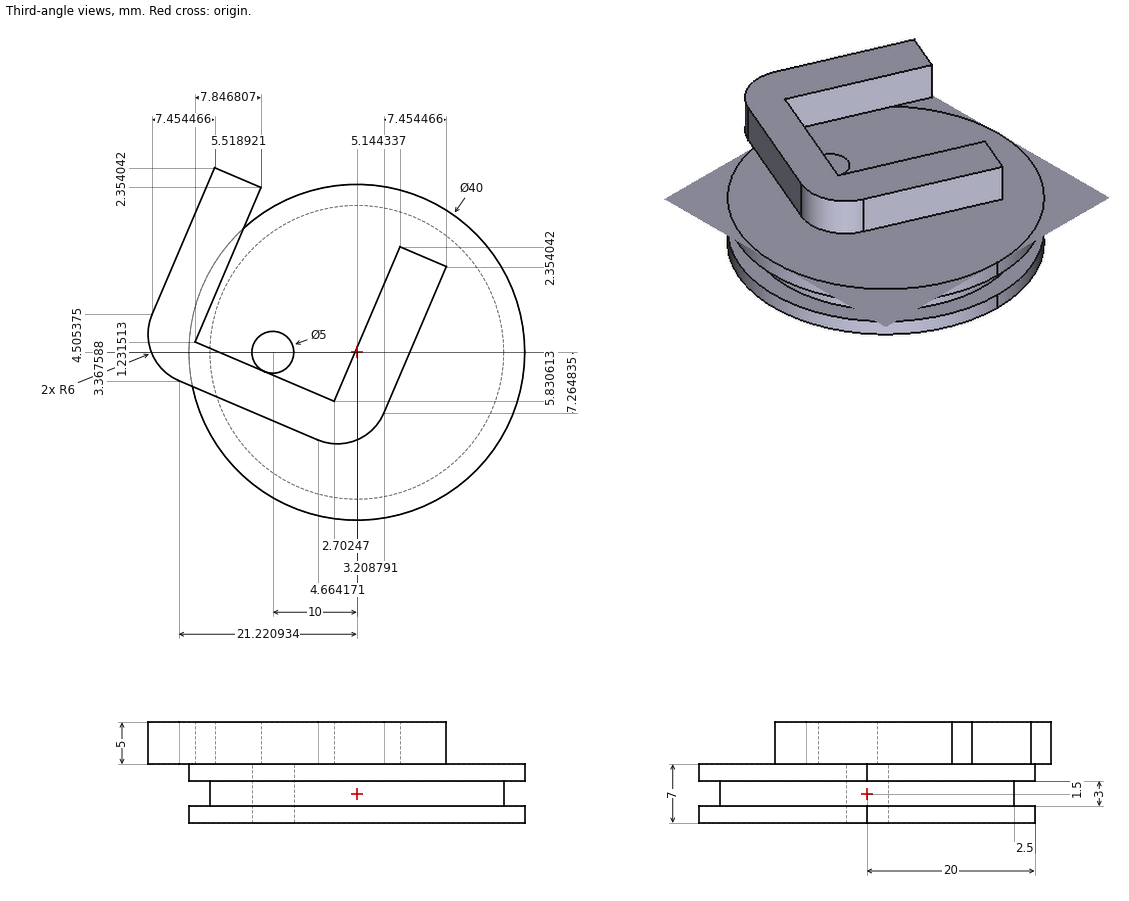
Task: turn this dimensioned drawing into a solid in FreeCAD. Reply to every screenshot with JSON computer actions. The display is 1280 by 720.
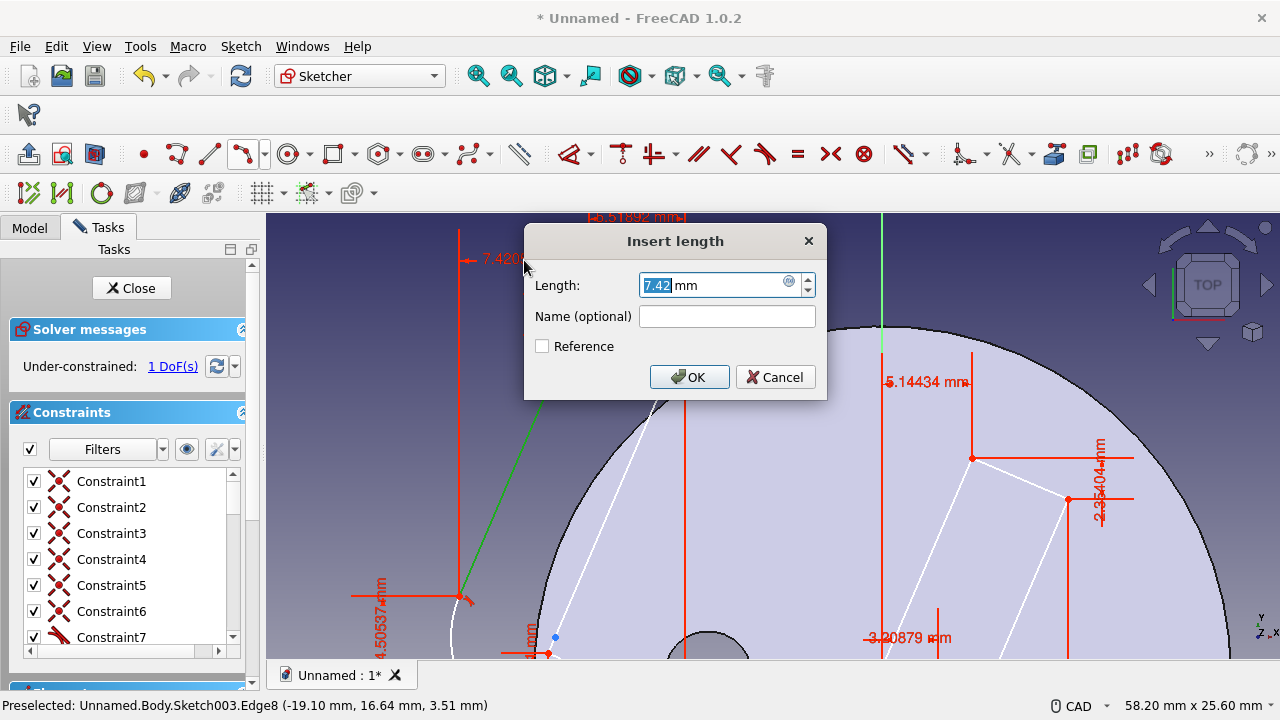
{"action": "type", "text": "7.454466"}
{"action": "key", "text": "Return"}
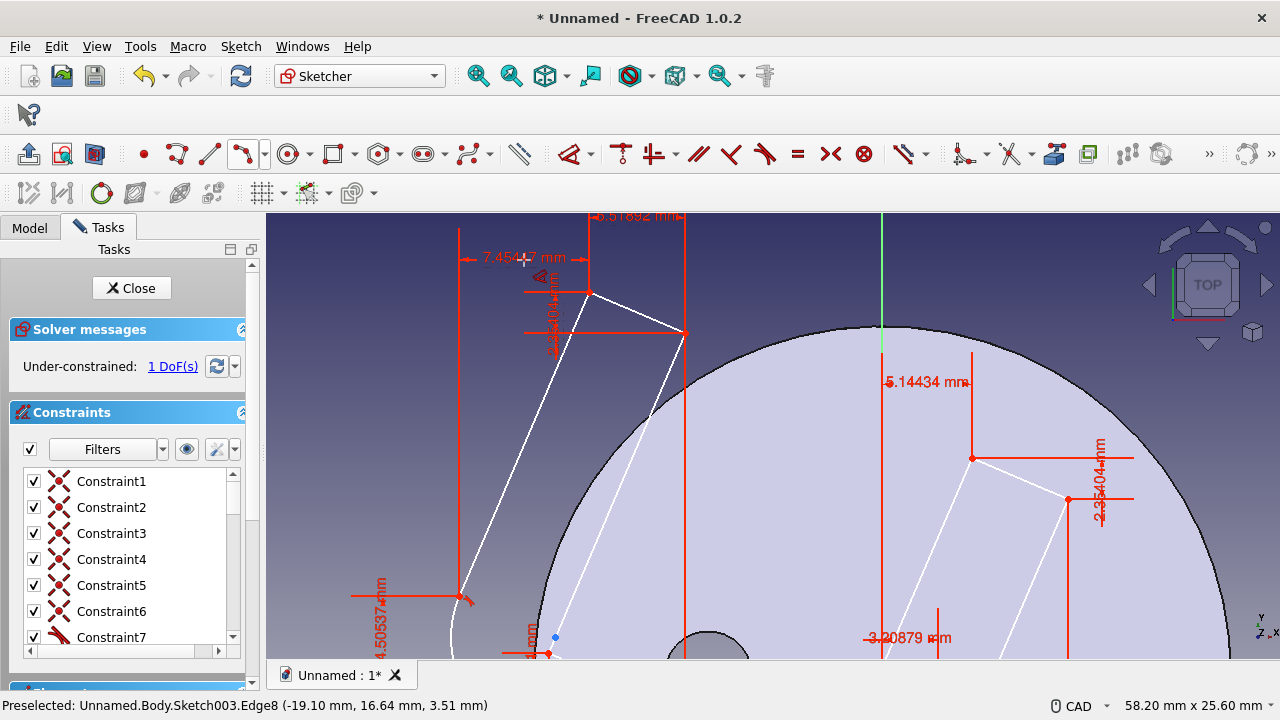
{"action": "scroll", "coordinate": [657, 323], "scroll_direction": "down", "scroll_amount": 4}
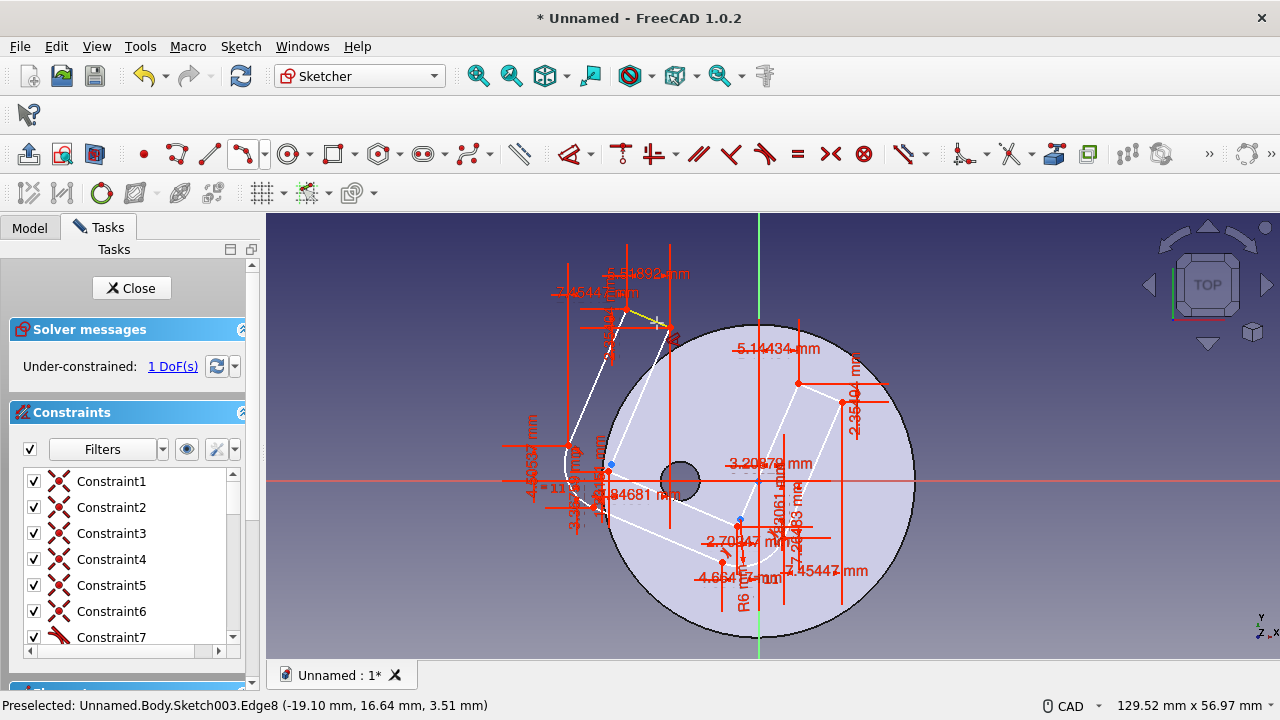
{"action": "left_click", "coordinate": [593, 508]}
{"action": "left_click", "coordinate": [638, 542]}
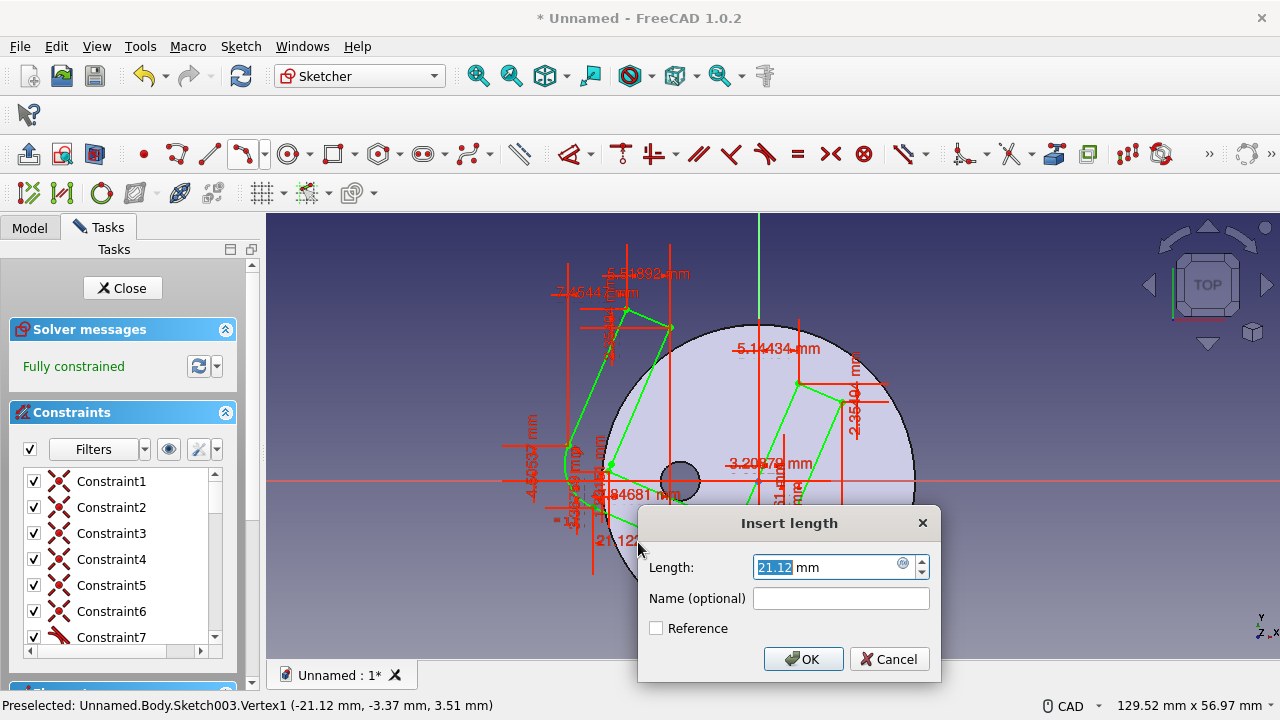
{"action": "type", "text": "21.220934"}
{"action": "key", "text": "Return"}
{"action": "key", "text": "Escape"}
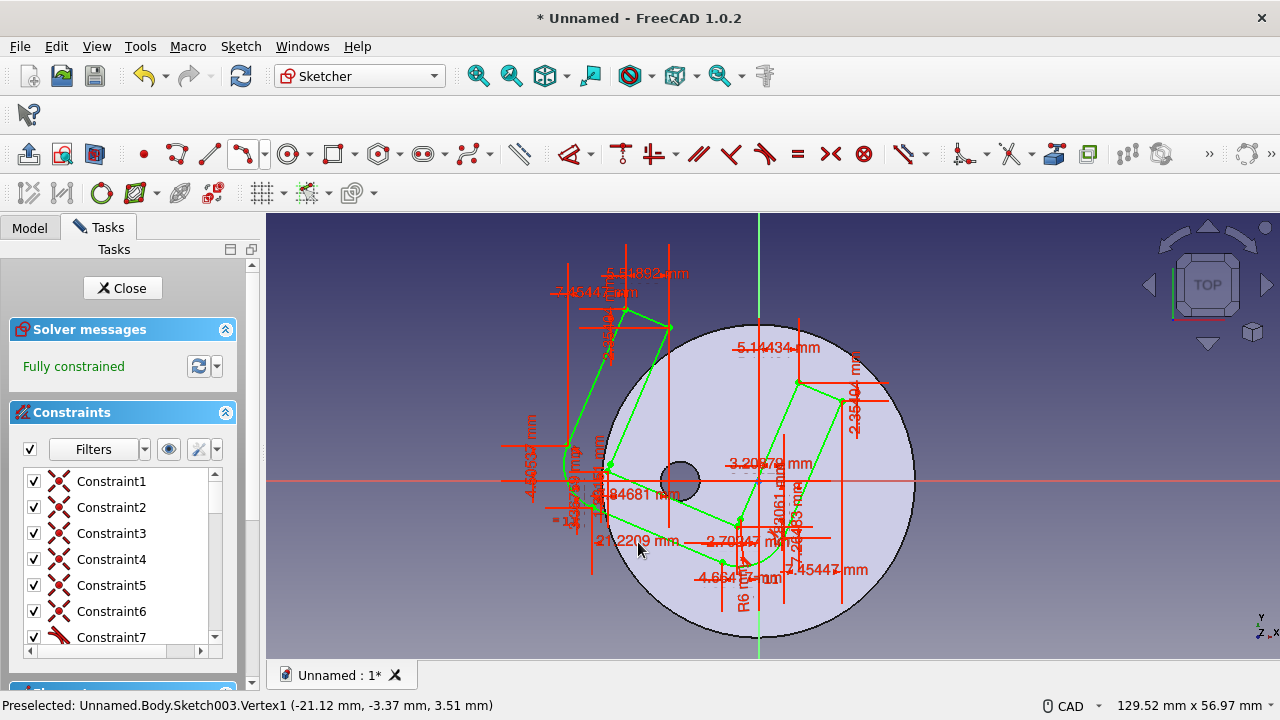
{"action": "left_click", "coordinate": [123, 288]}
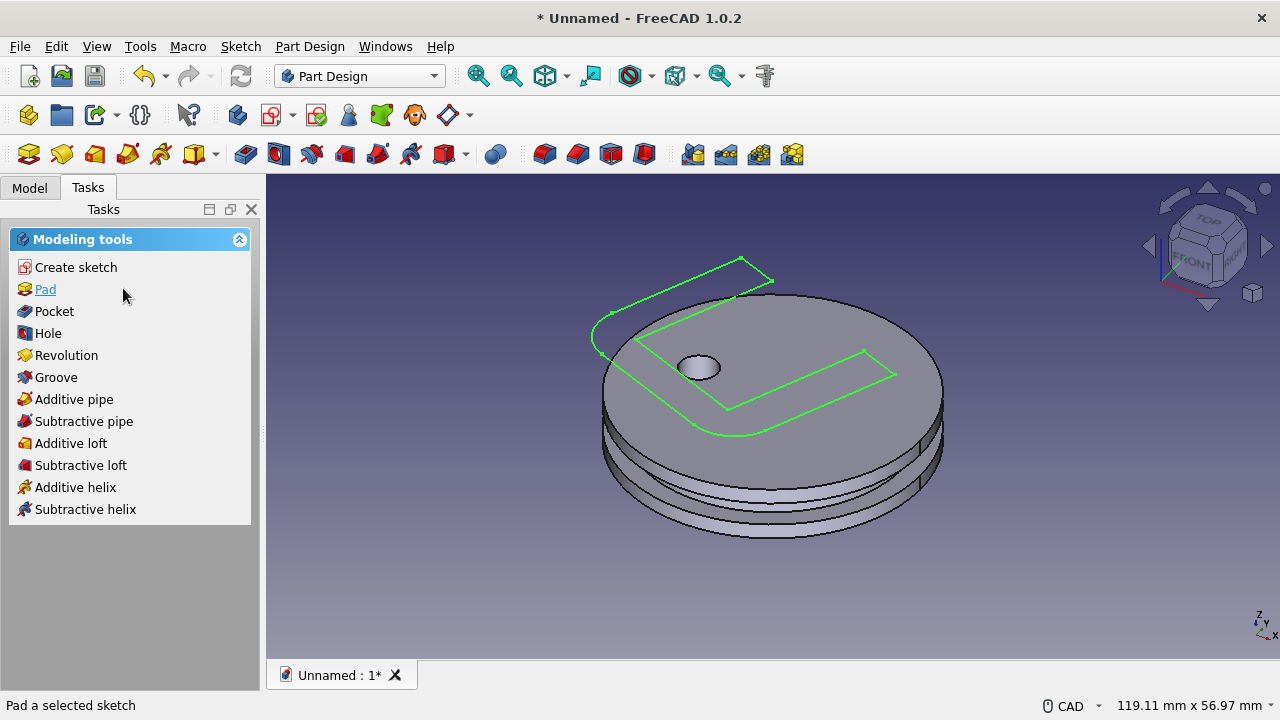
{"action": "left_click", "coordinate": [29, 154]}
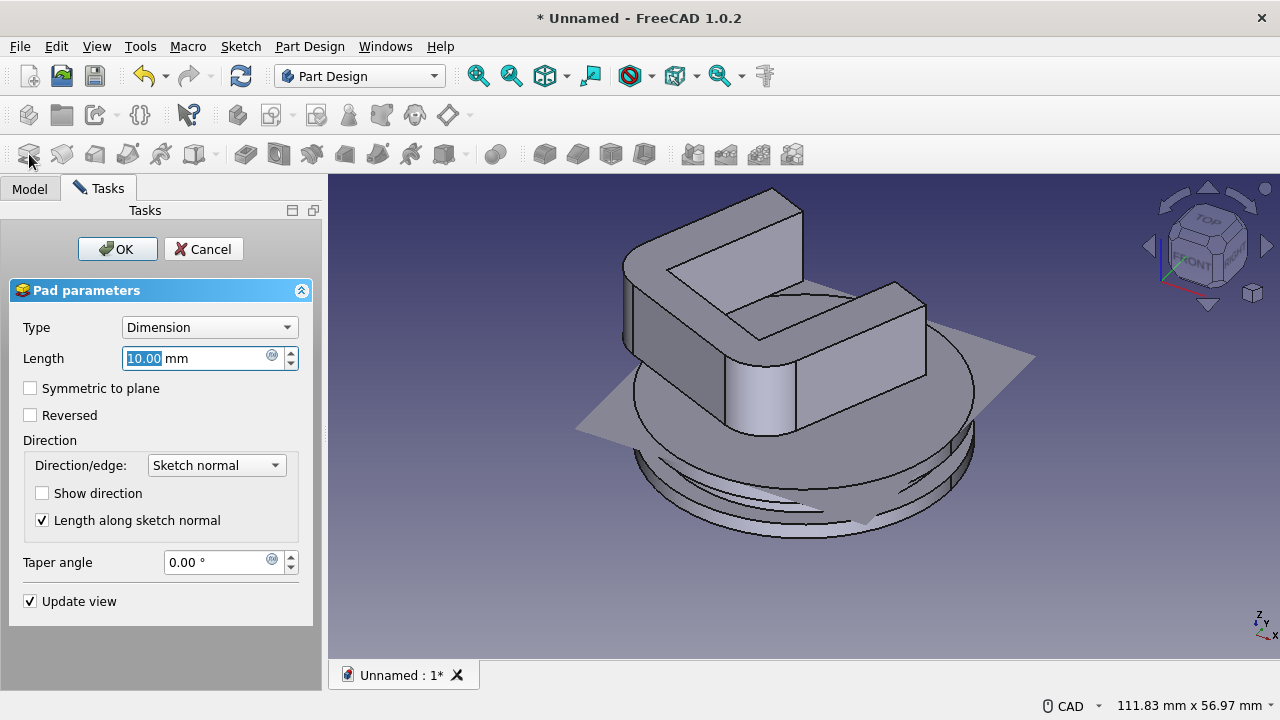
{"action": "type", "text": "5"}
{"action": "key", "text": "Tab"}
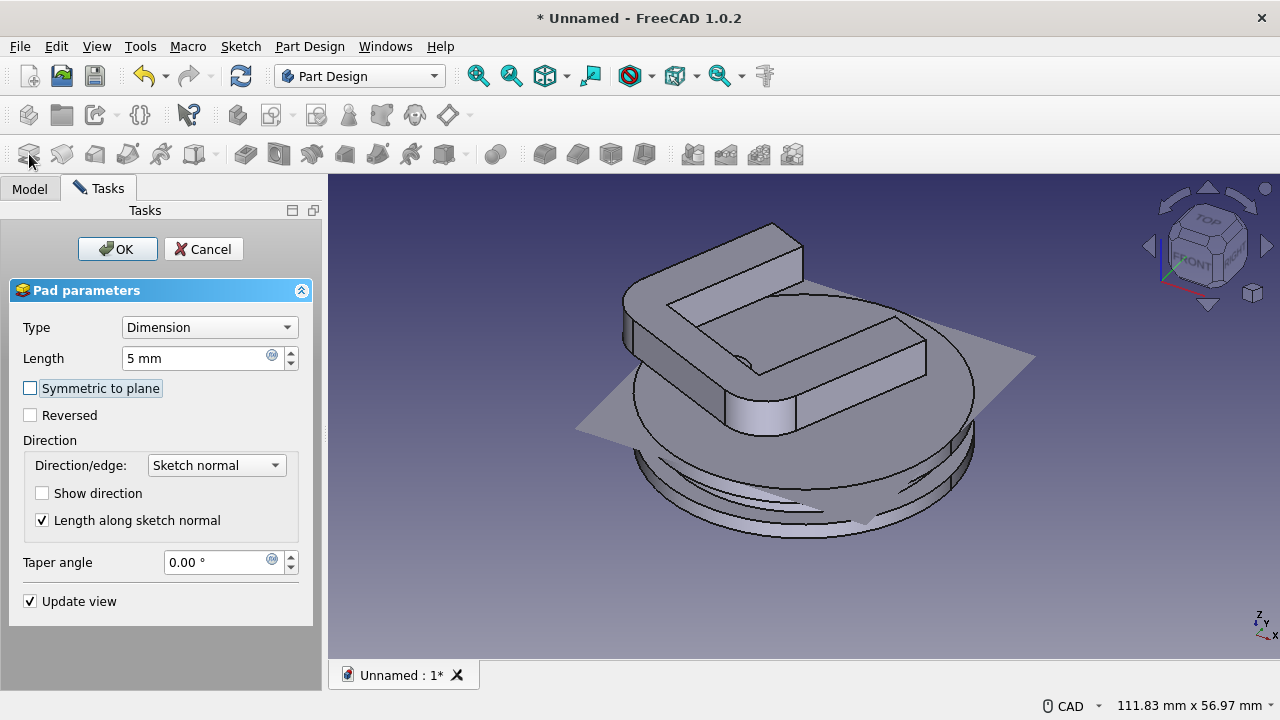
{"action": "left_click", "coordinate": [118, 249]}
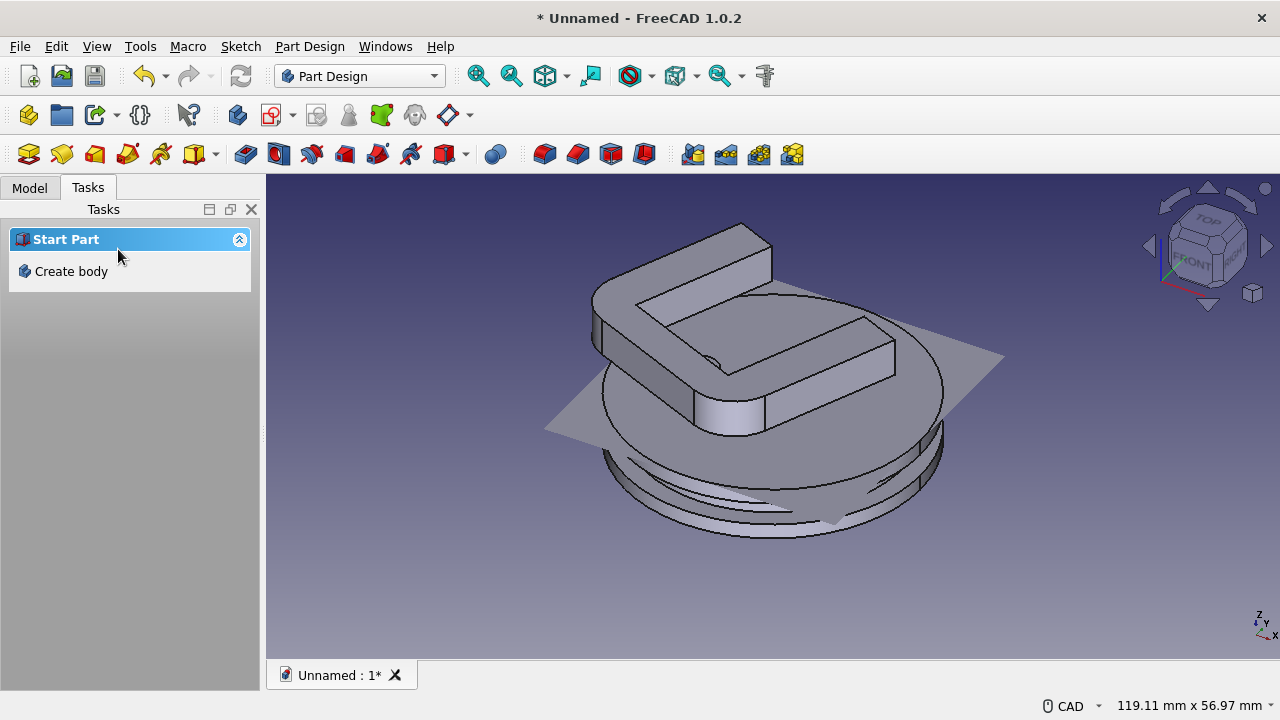
{"action": "key", "text": "0"}